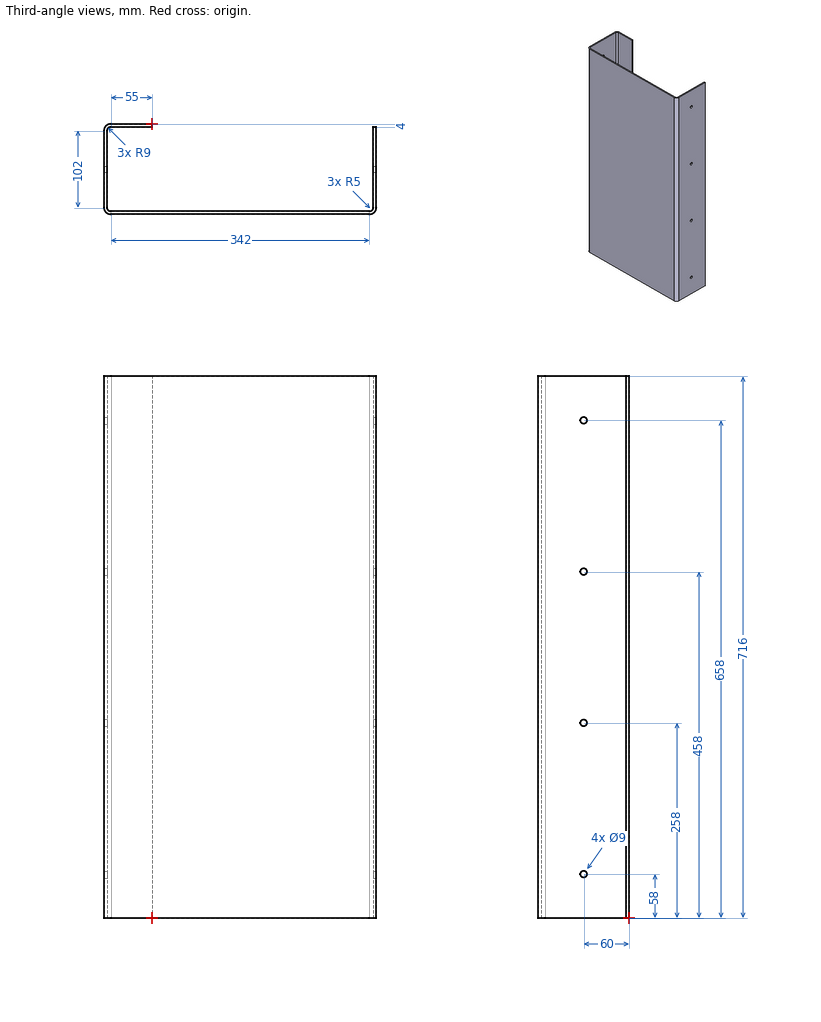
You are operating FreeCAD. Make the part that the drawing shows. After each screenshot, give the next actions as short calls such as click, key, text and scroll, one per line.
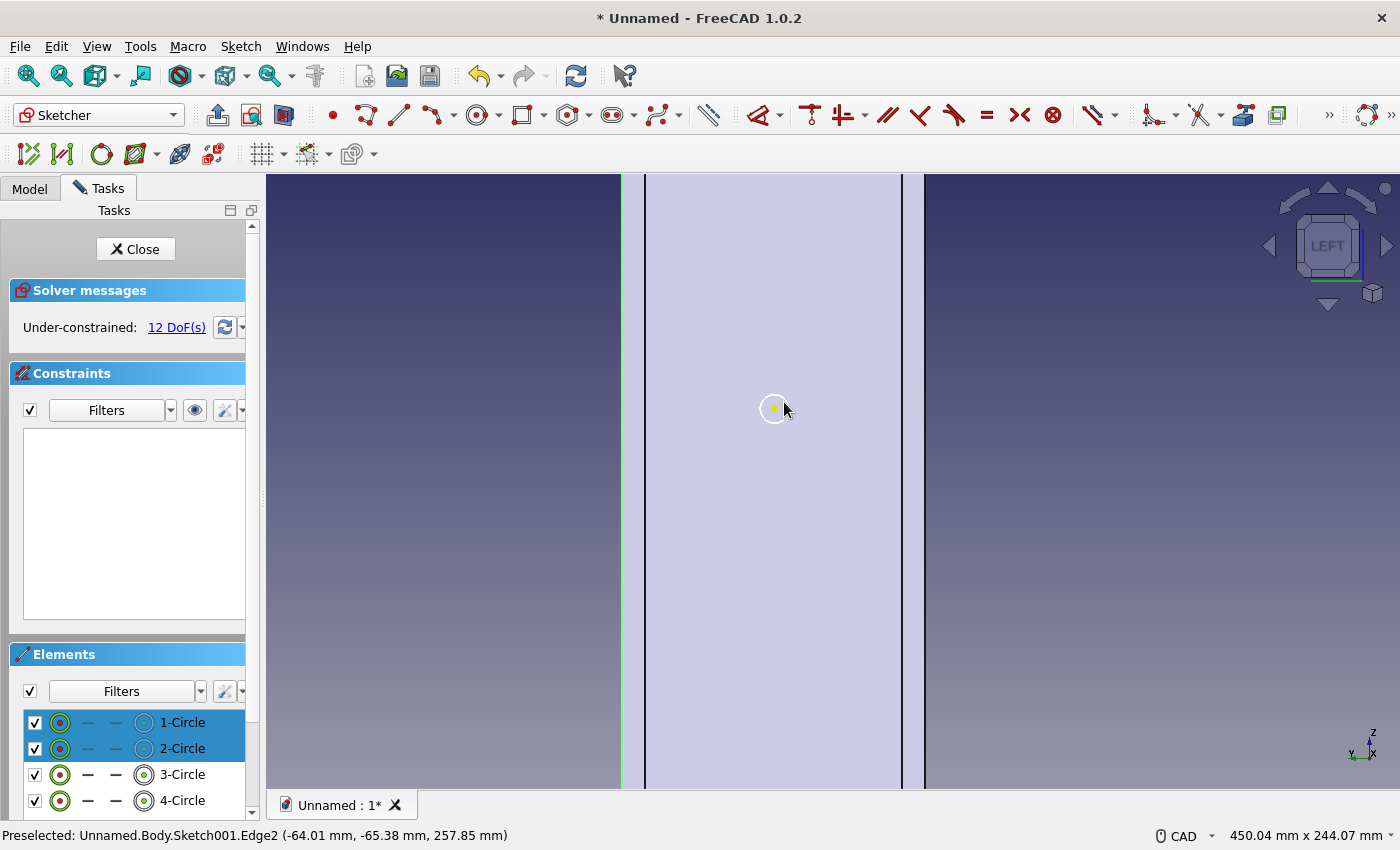
click(784, 399)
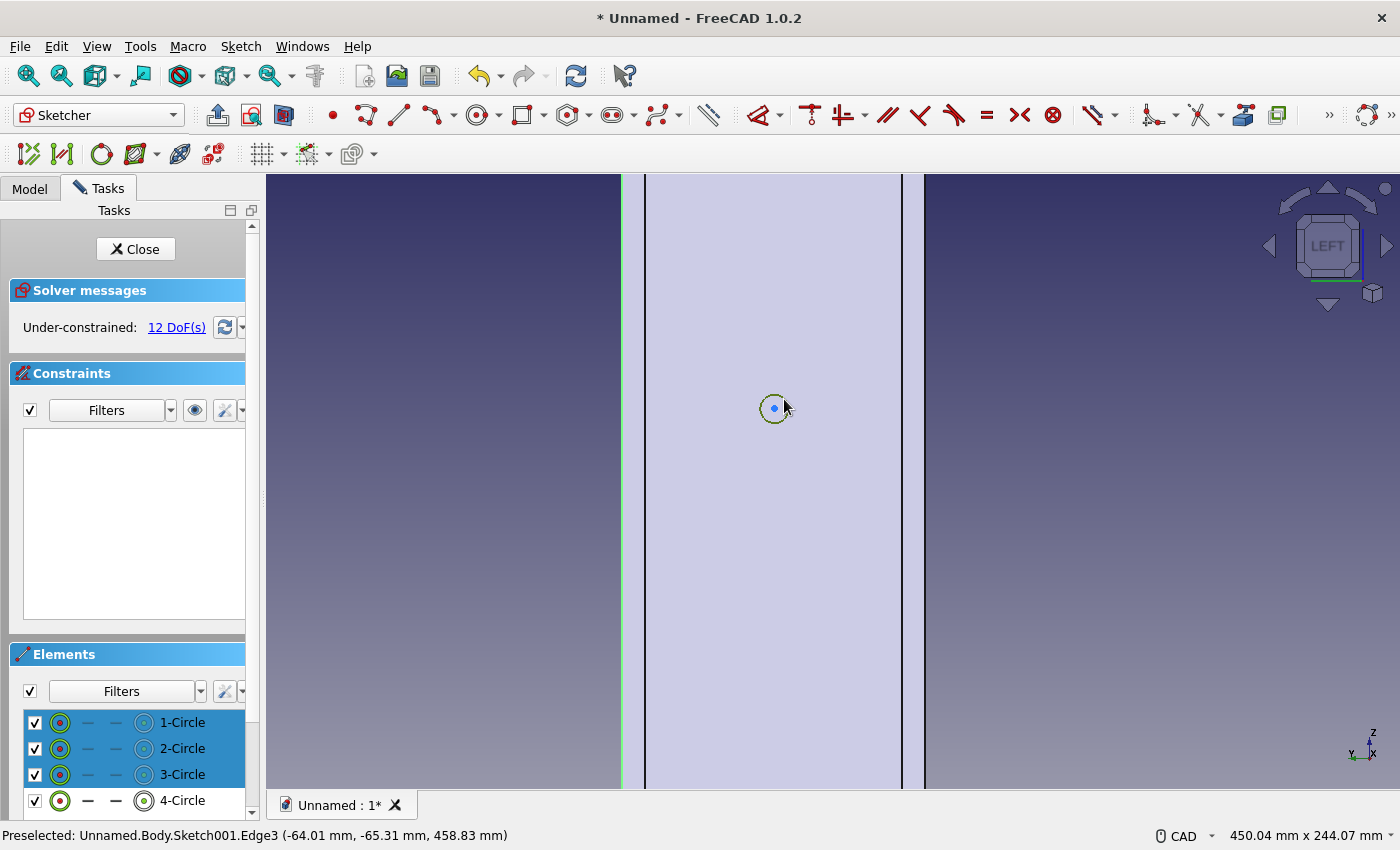
scroll(784, 402, down, 7)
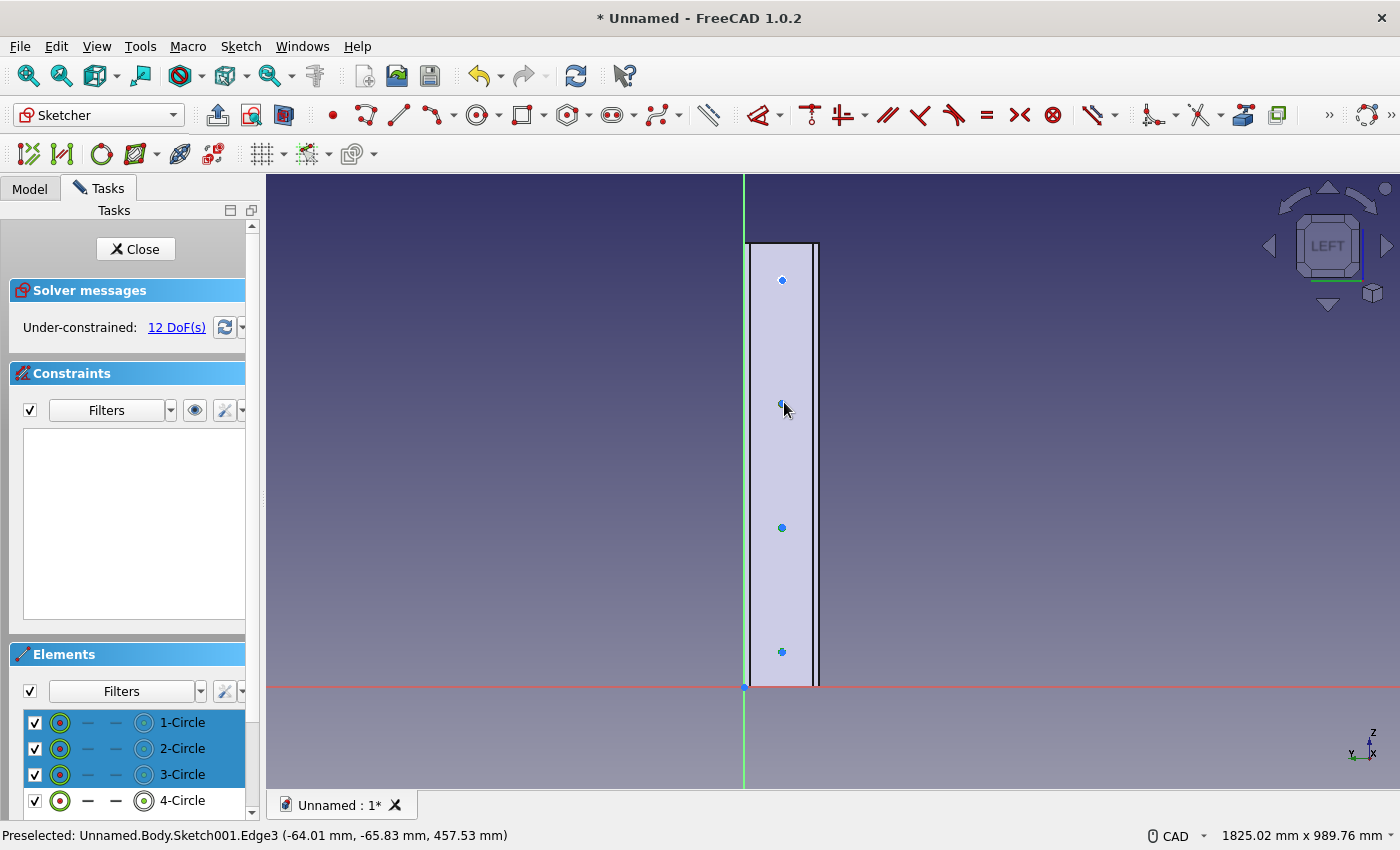
scroll(785, 277, up, 7)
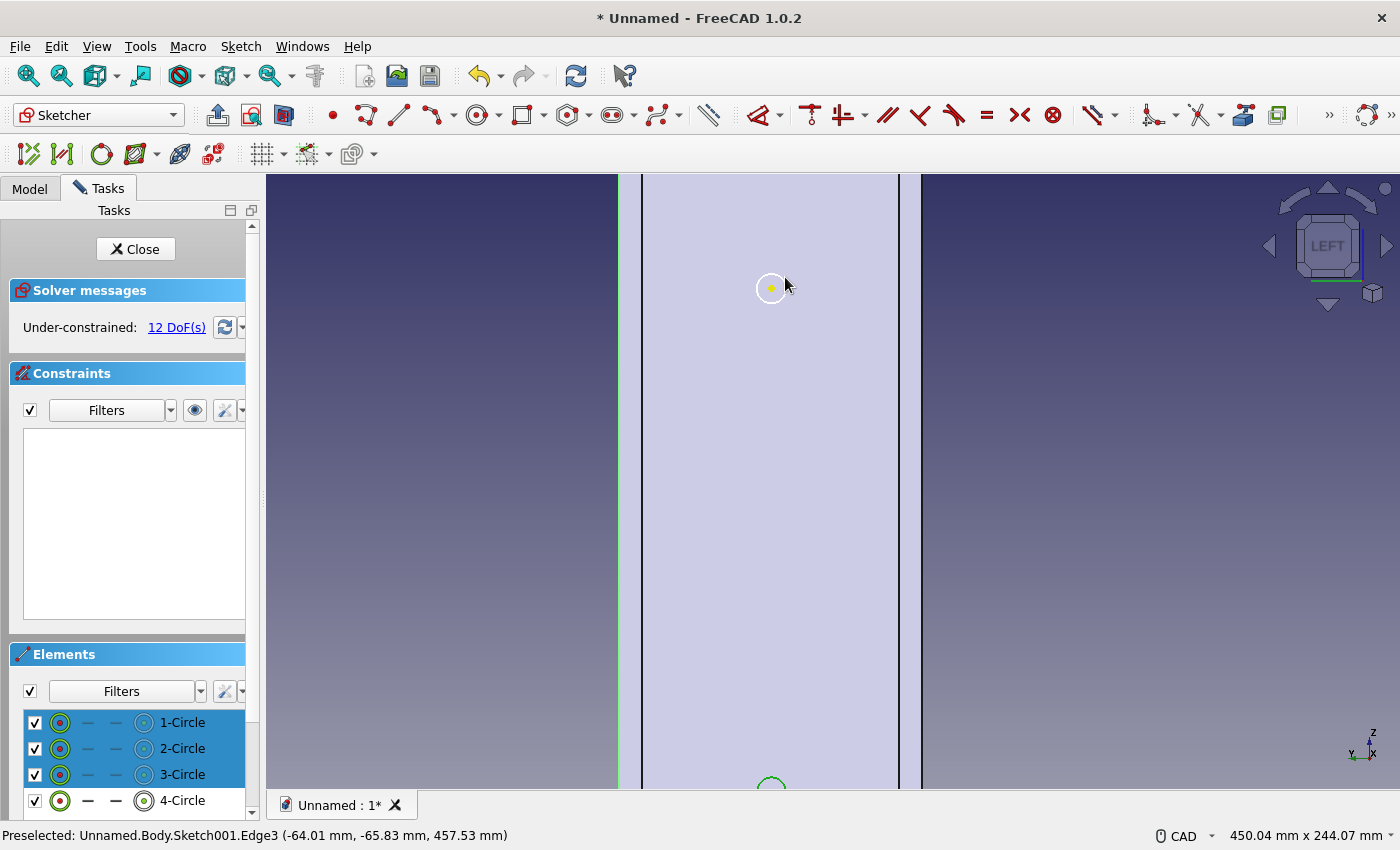
click(782, 278)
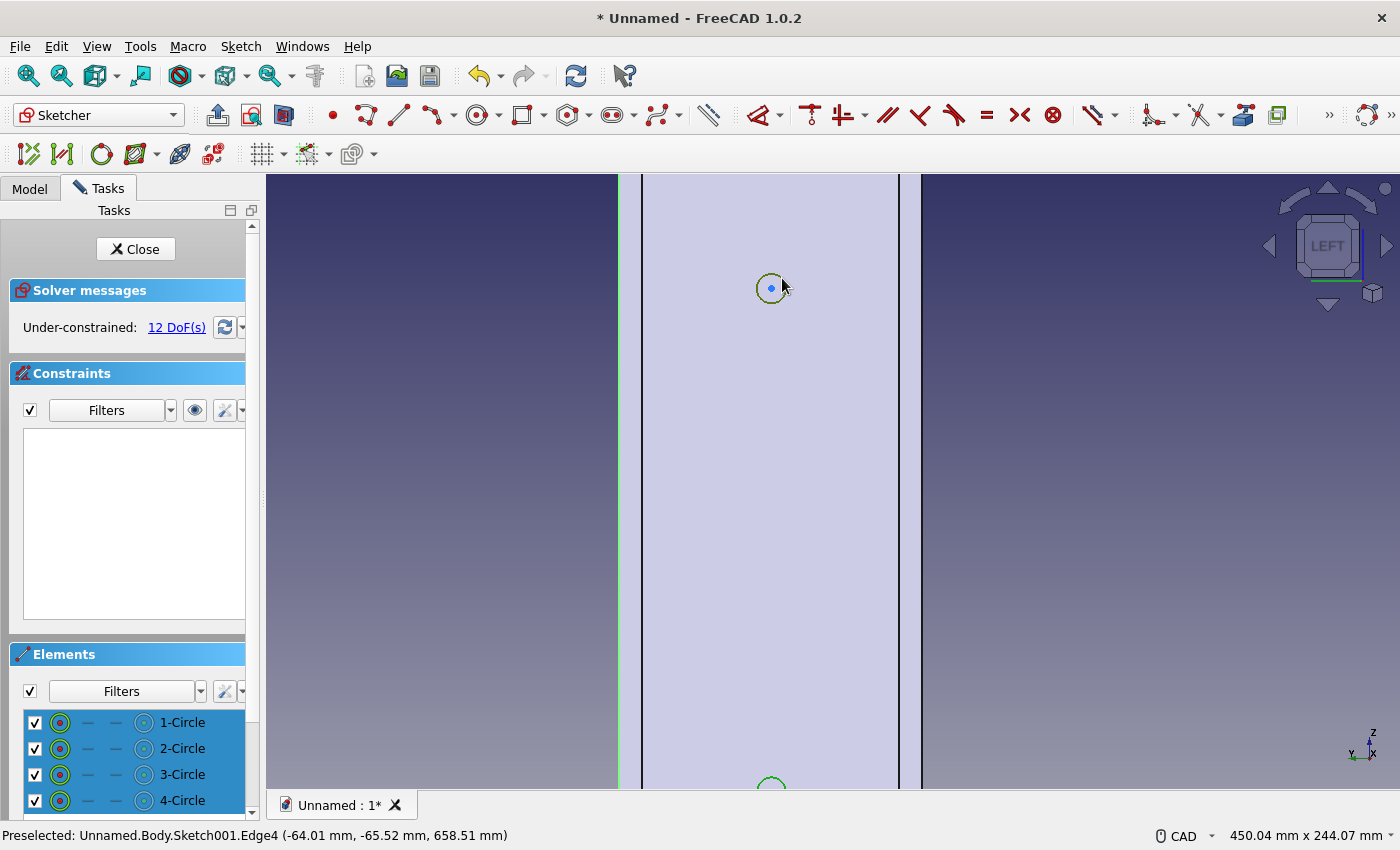
click(987, 116)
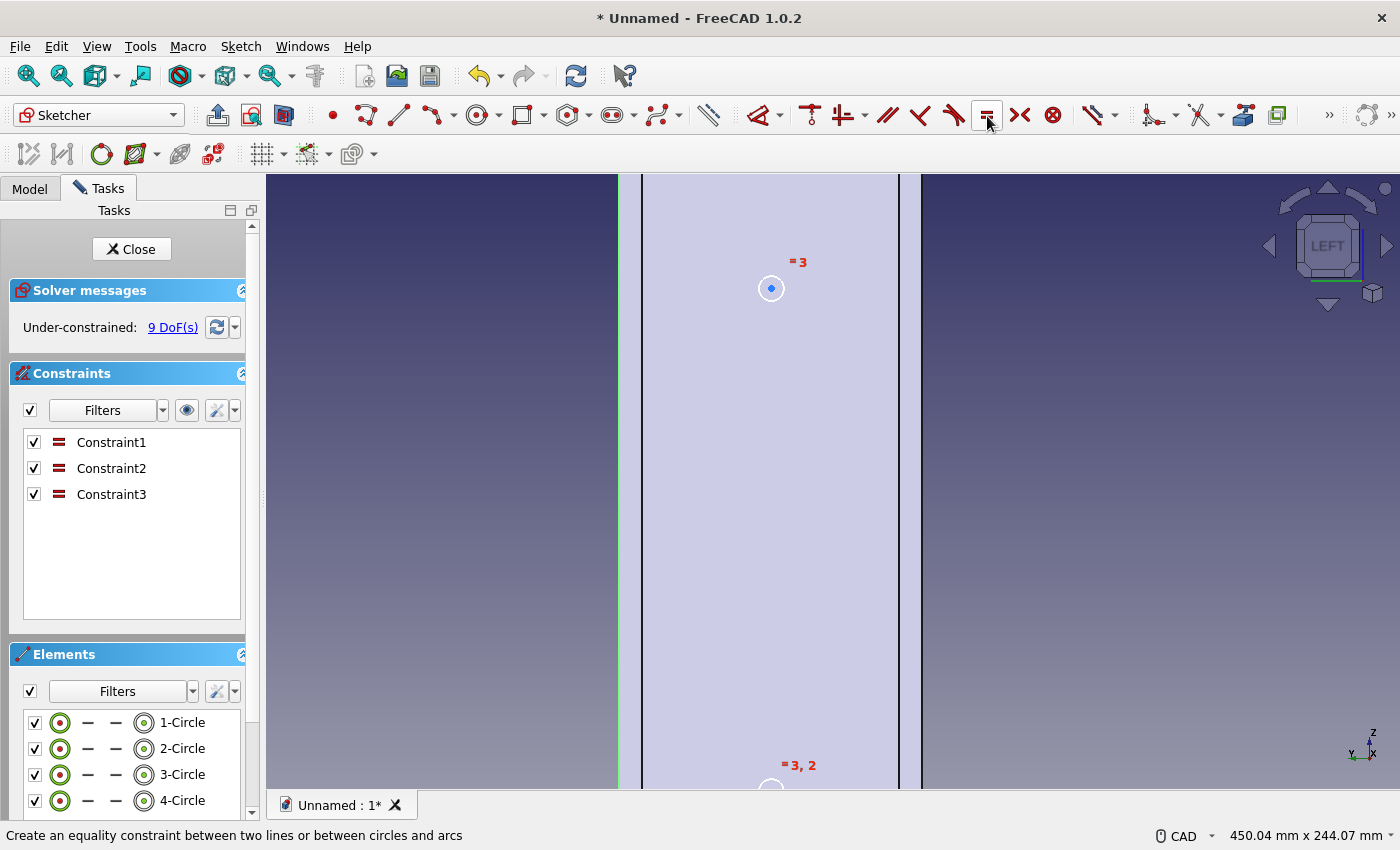
scroll(785, 277, down, 7)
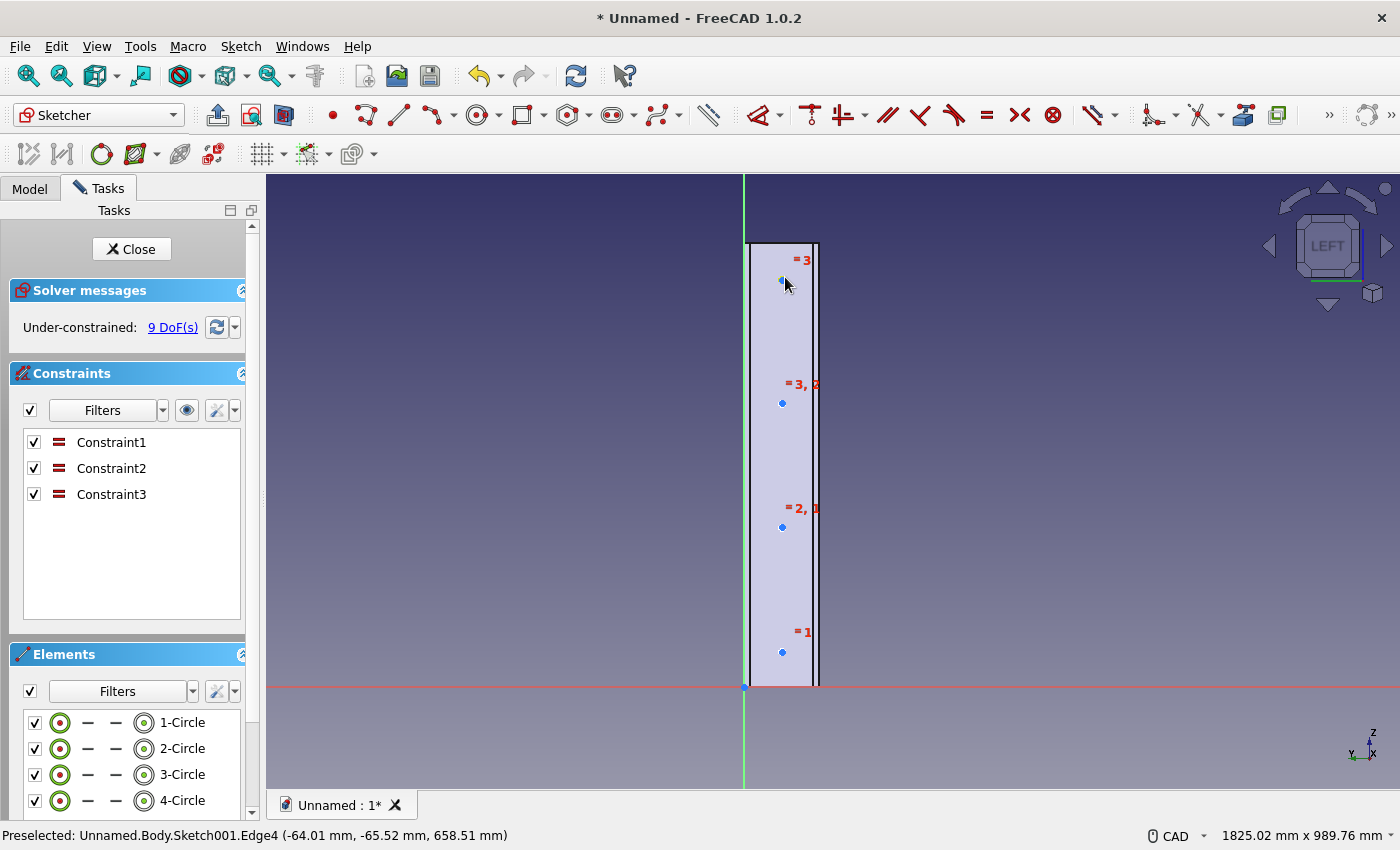
click(782, 652)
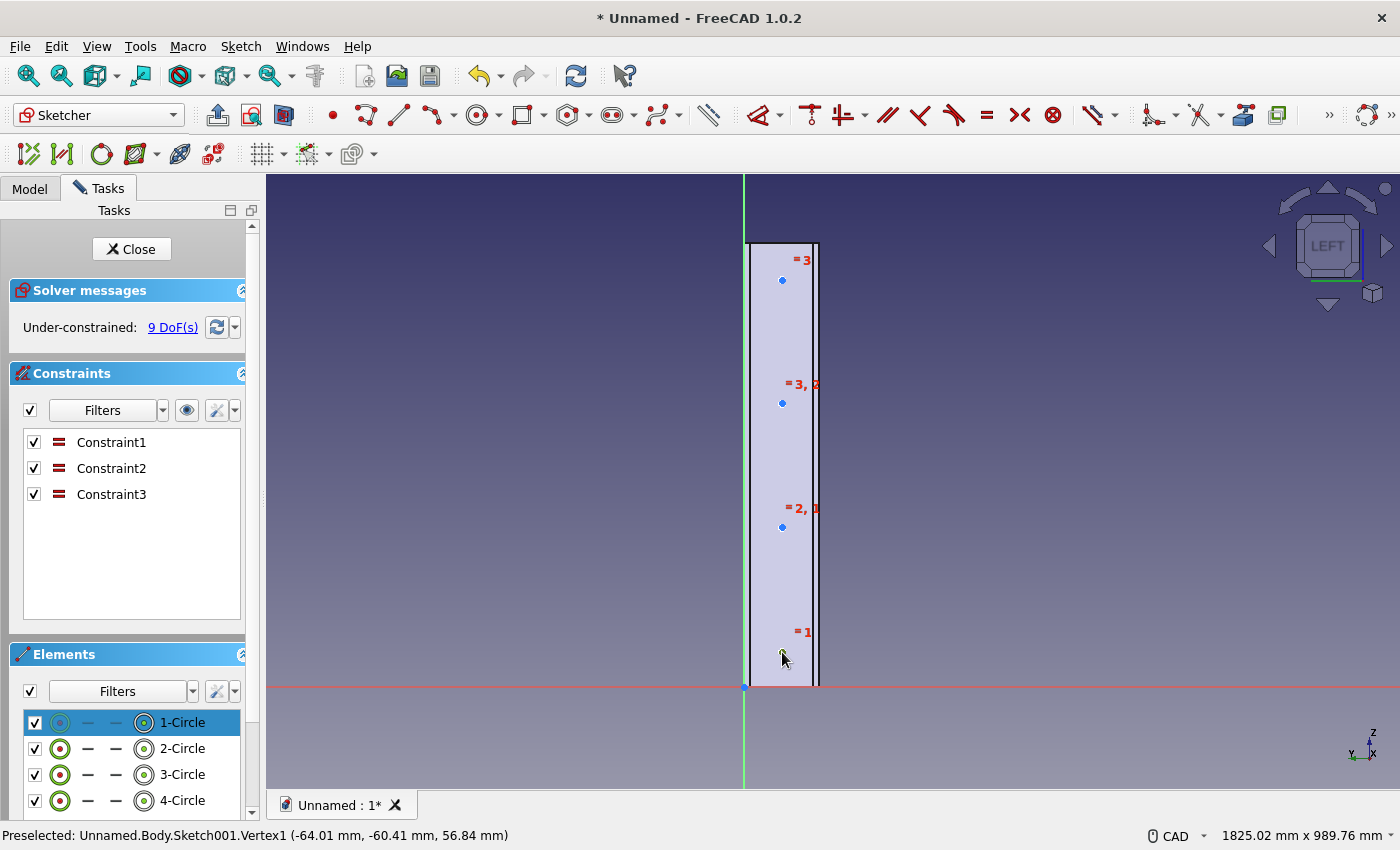
click(782, 528)